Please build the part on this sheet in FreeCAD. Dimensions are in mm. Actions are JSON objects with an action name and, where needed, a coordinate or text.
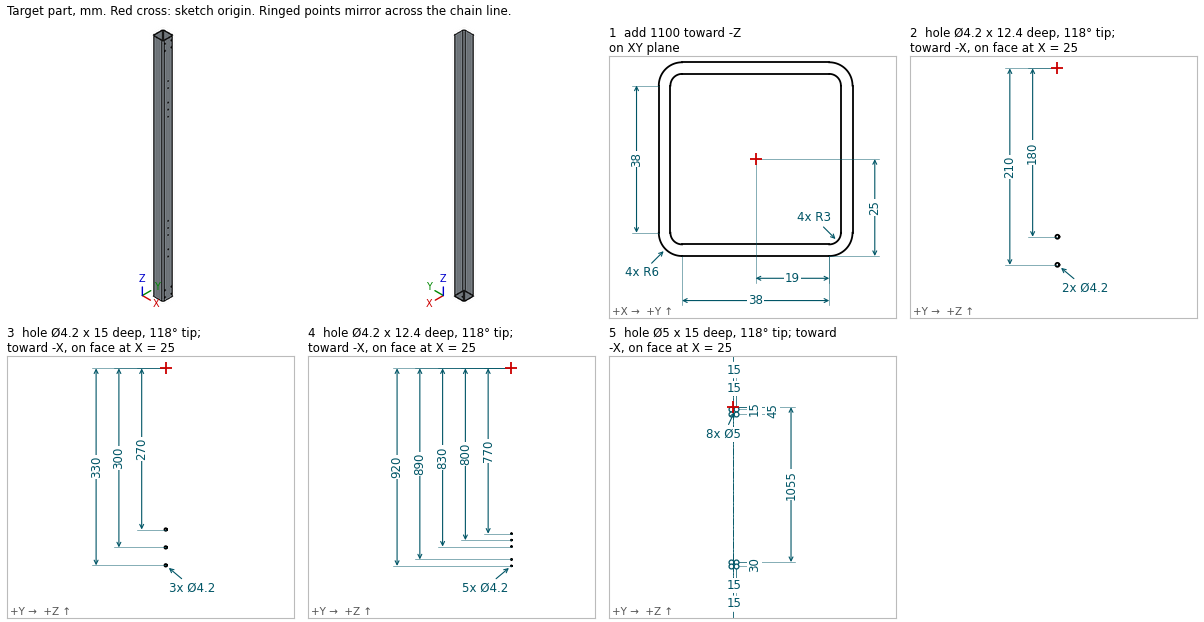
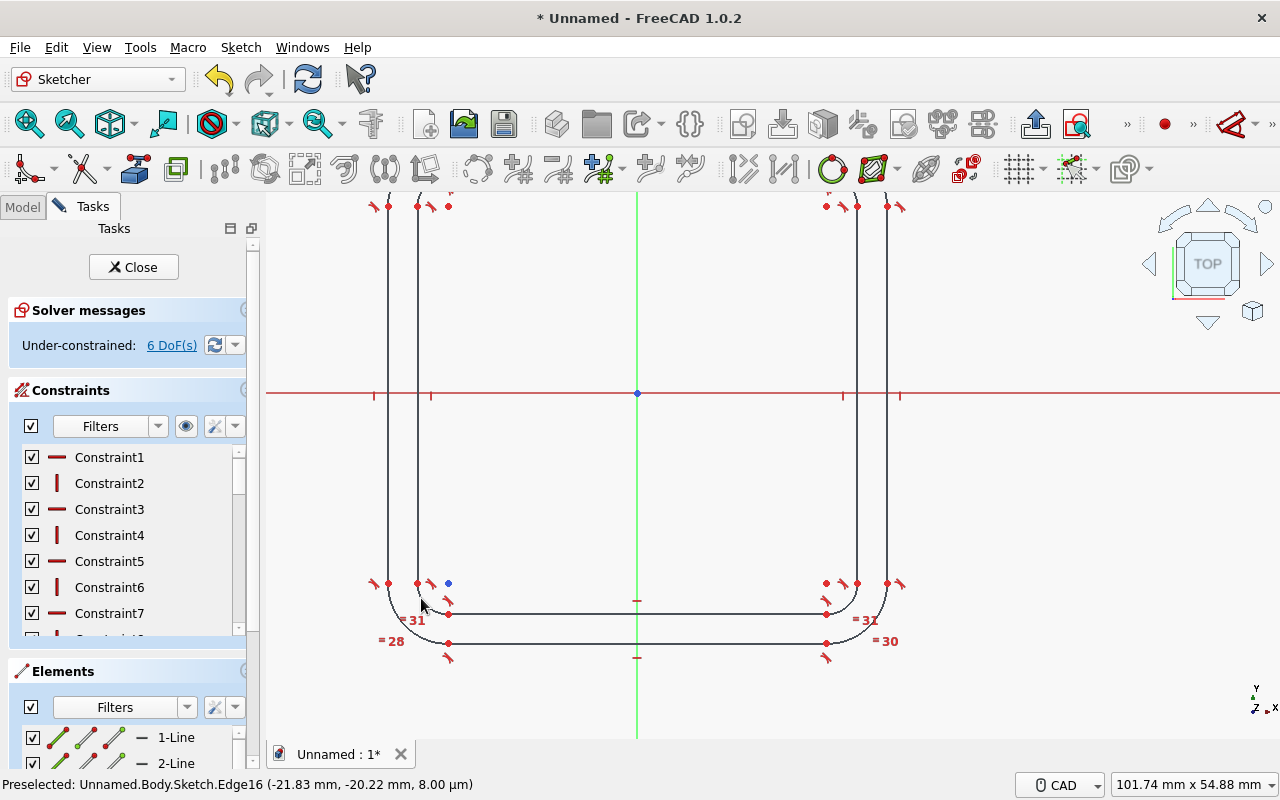
{"action": "left_click", "coordinate": [395, 611]}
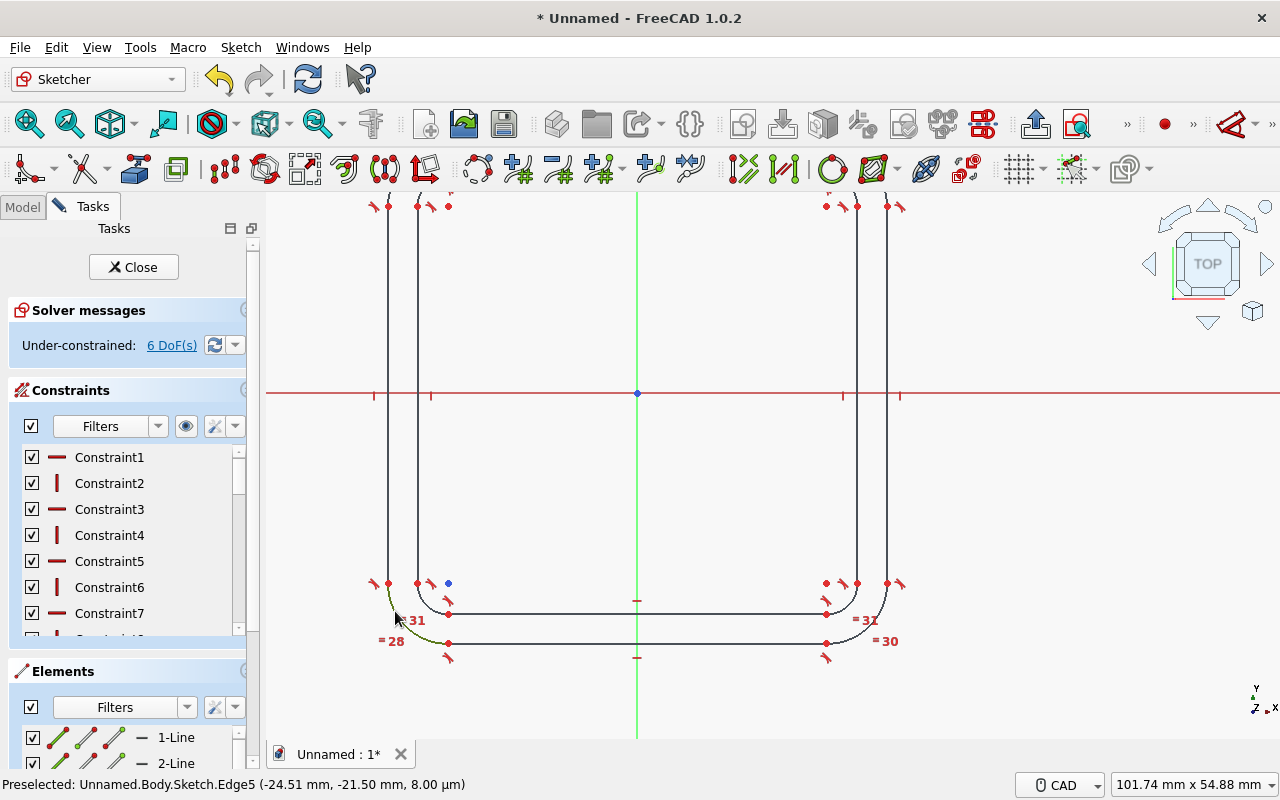
{"action": "left_click", "coordinate": [1258, 124]}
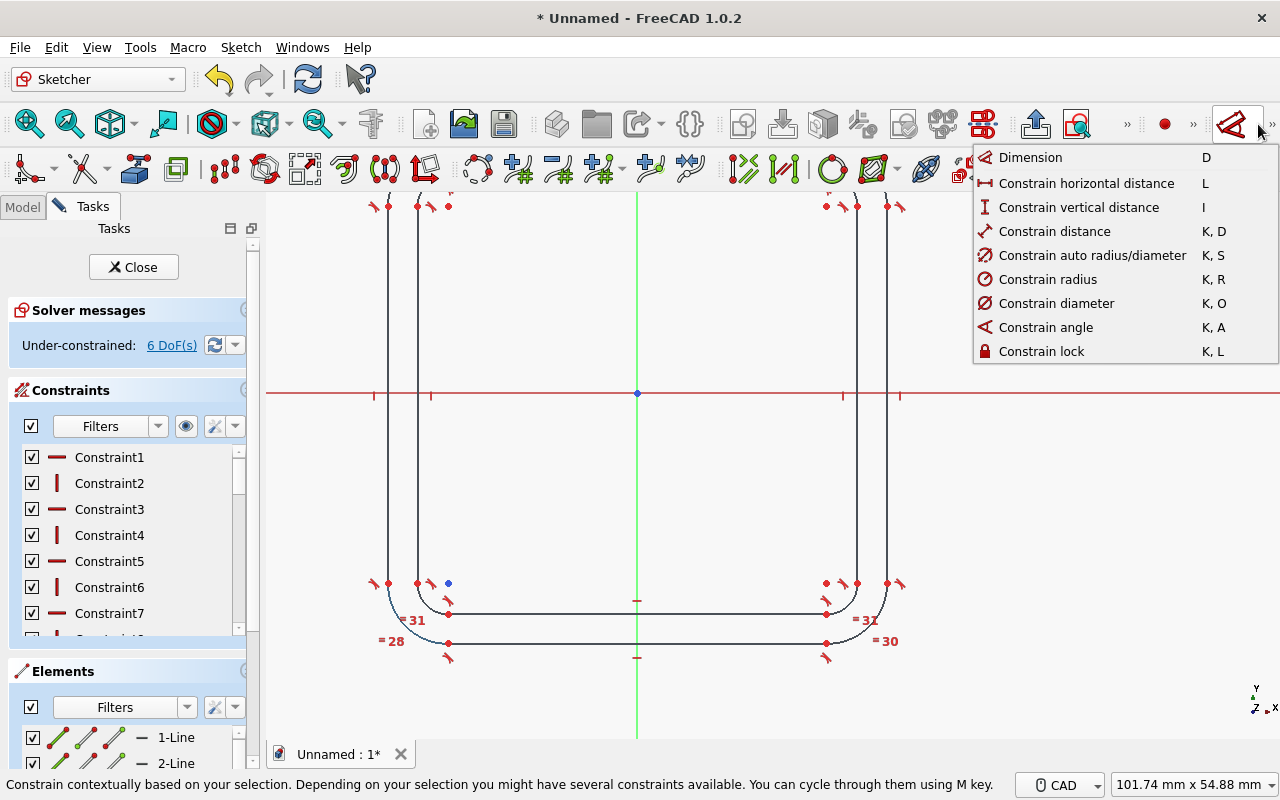
{"action": "left_click", "coordinate": [1126, 279]}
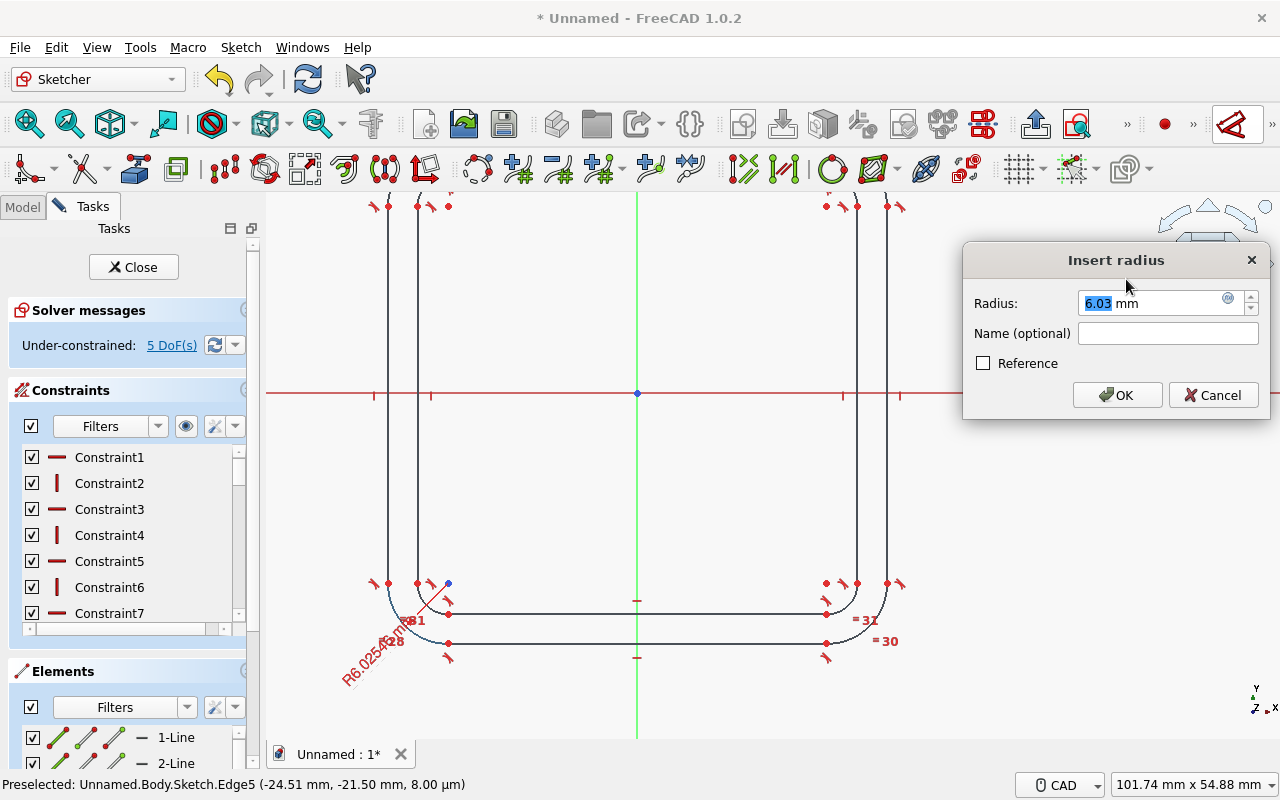
{"action": "type", "text": "6"}
{"action": "key", "text": "Return"}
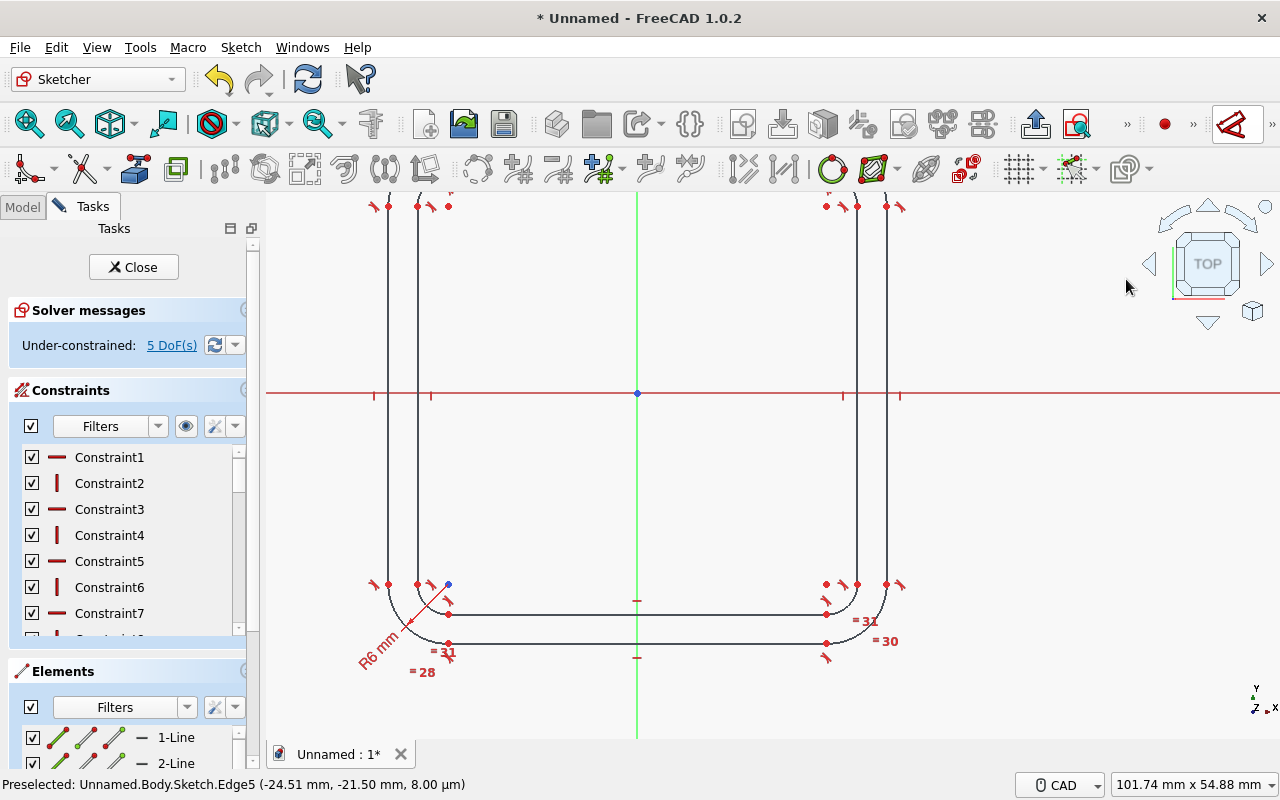
{"action": "scroll", "coordinate": [841, 611], "scroll_direction": "up", "scroll_amount": 2}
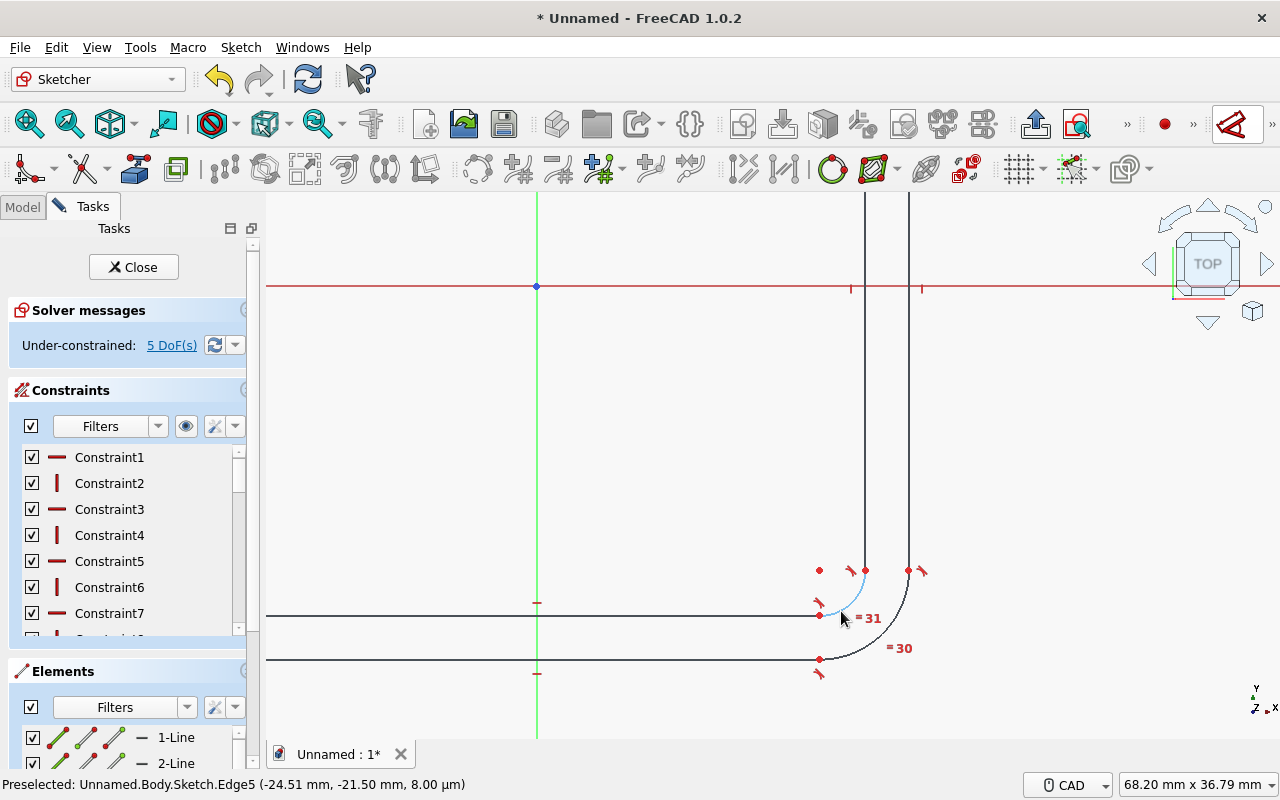
{"action": "left_click", "coordinate": [840, 611]}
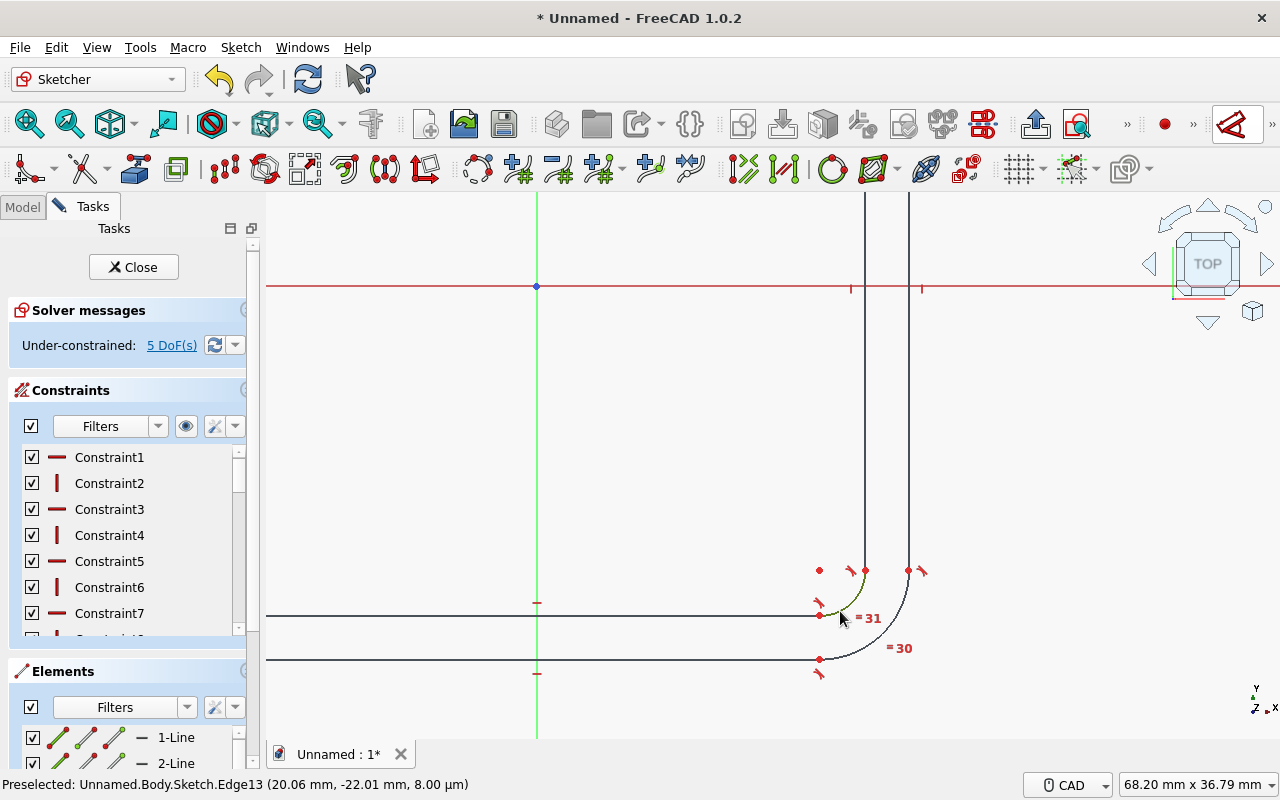
{"action": "left_click", "coordinate": [1258, 124]}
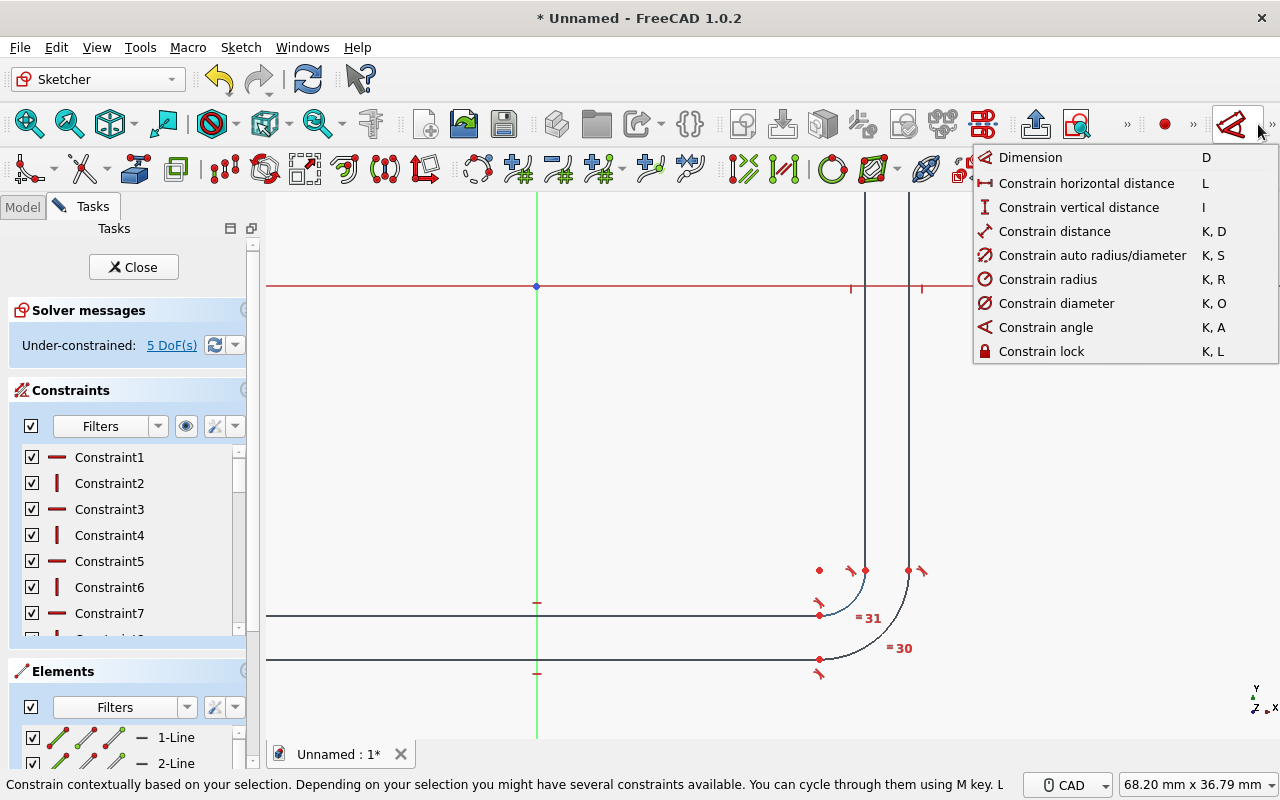
{"action": "left_click", "coordinate": [1126, 279]}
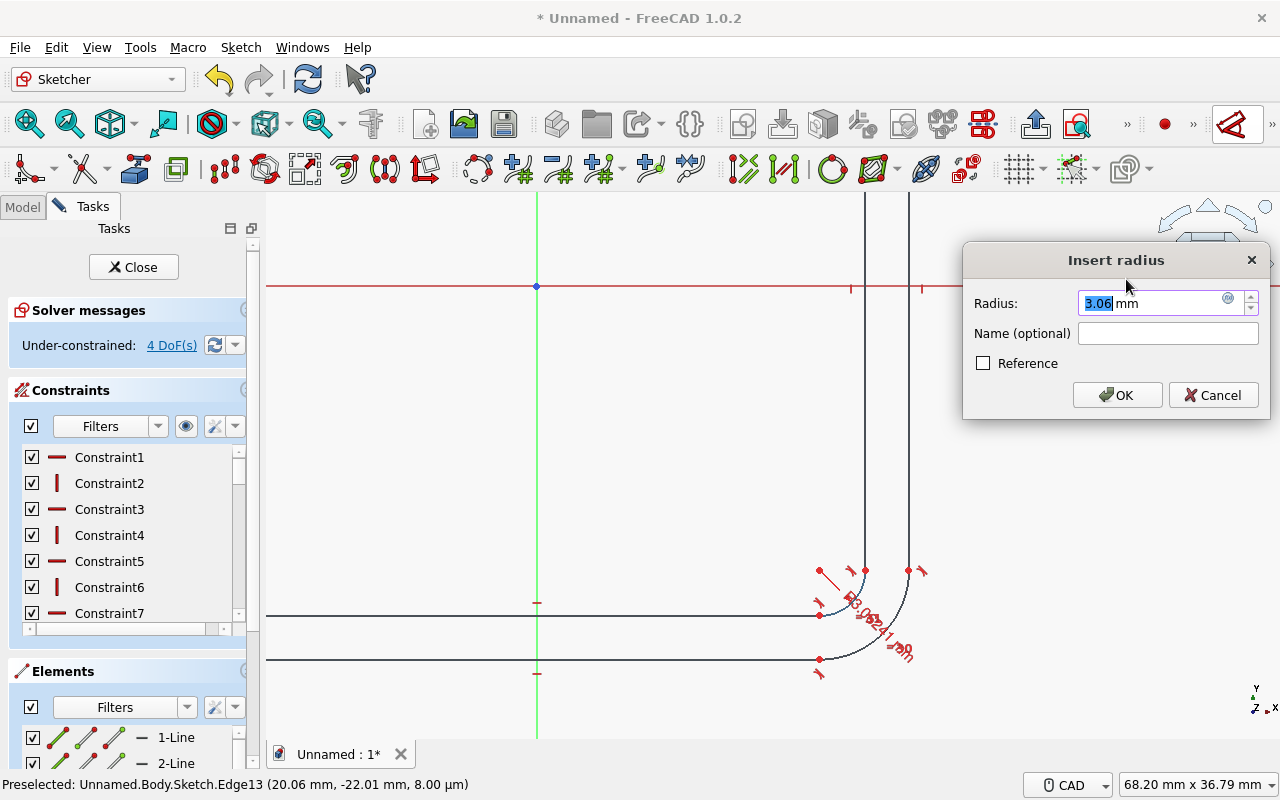
{"action": "type", "text": "3"}
{"action": "key", "text": "Return"}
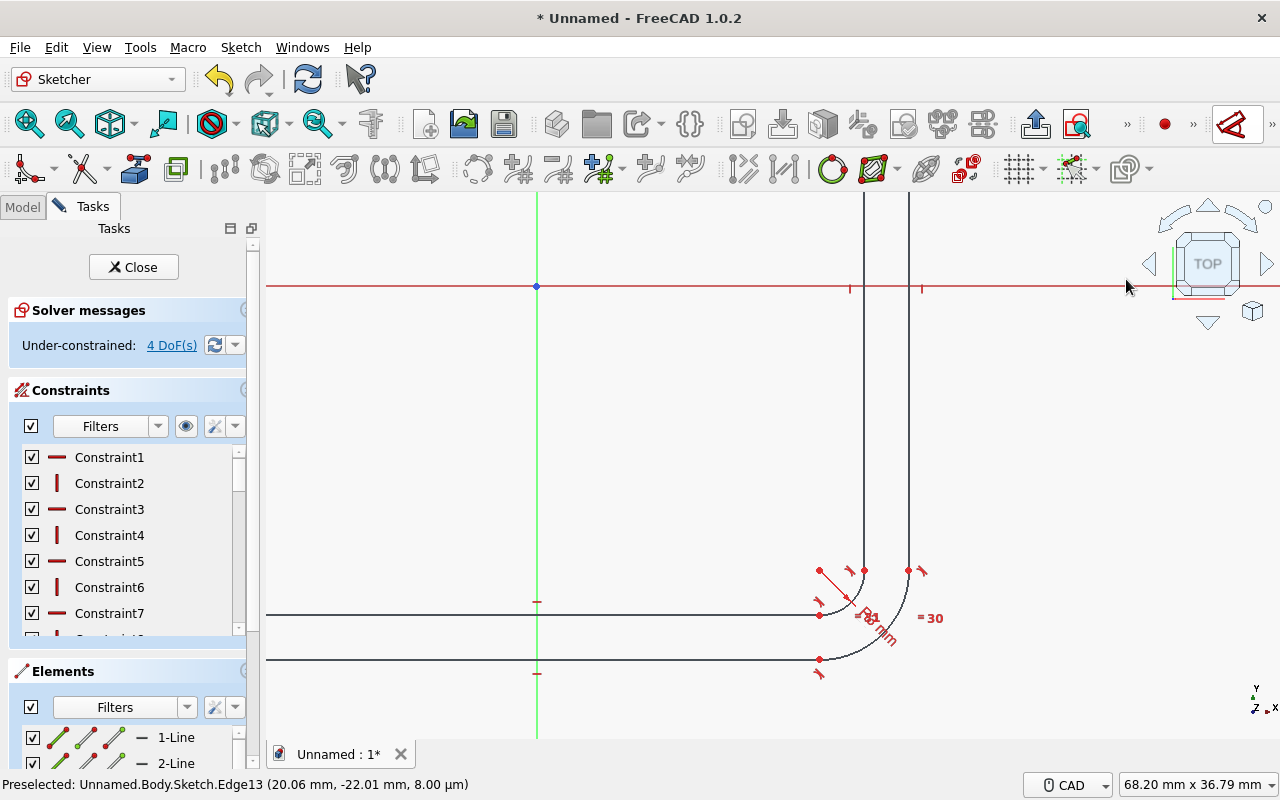
{"action": "left_click", "coordinate": [650, 660]}